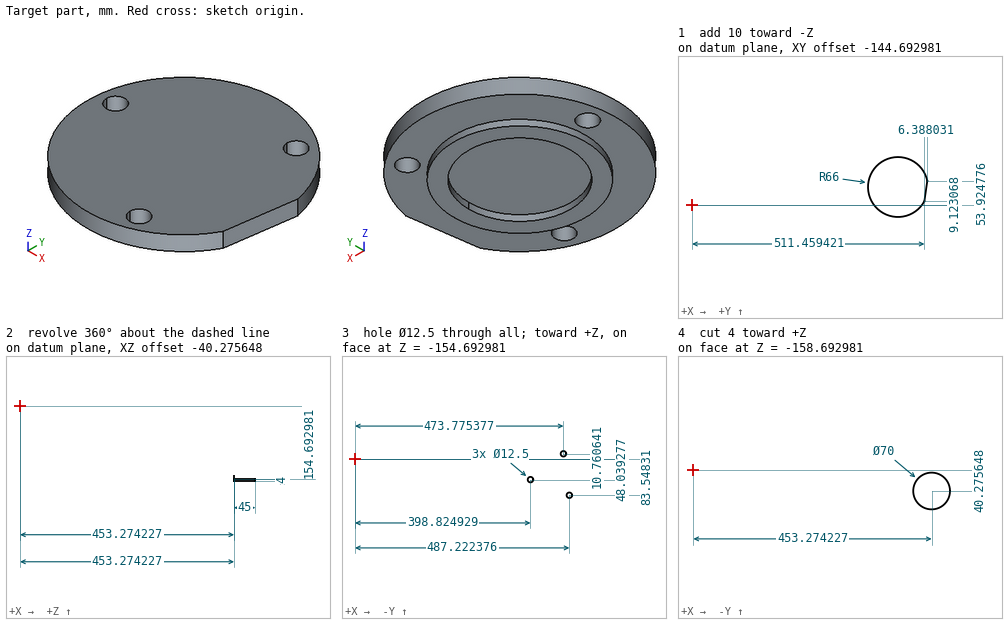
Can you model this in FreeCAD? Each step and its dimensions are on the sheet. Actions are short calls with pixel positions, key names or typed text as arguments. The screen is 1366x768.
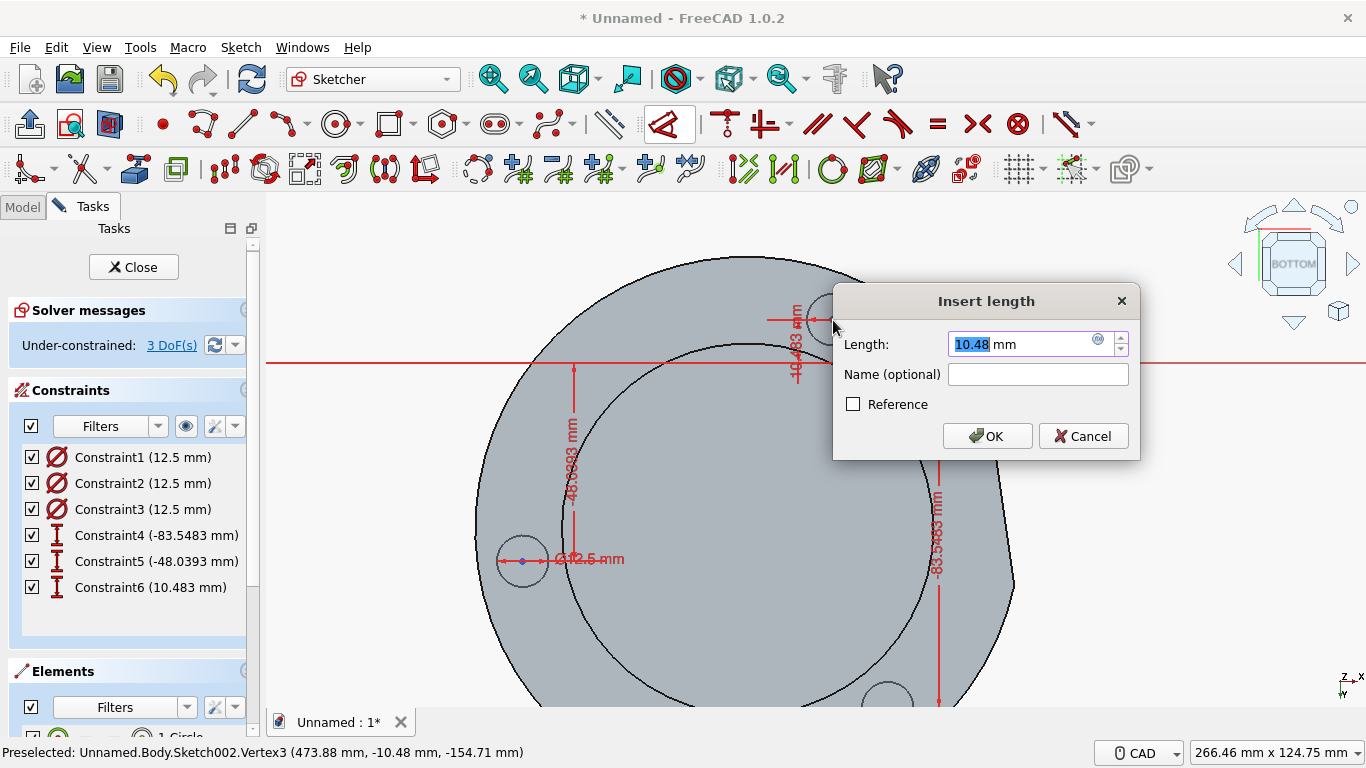
text(10.760641)
key(Return)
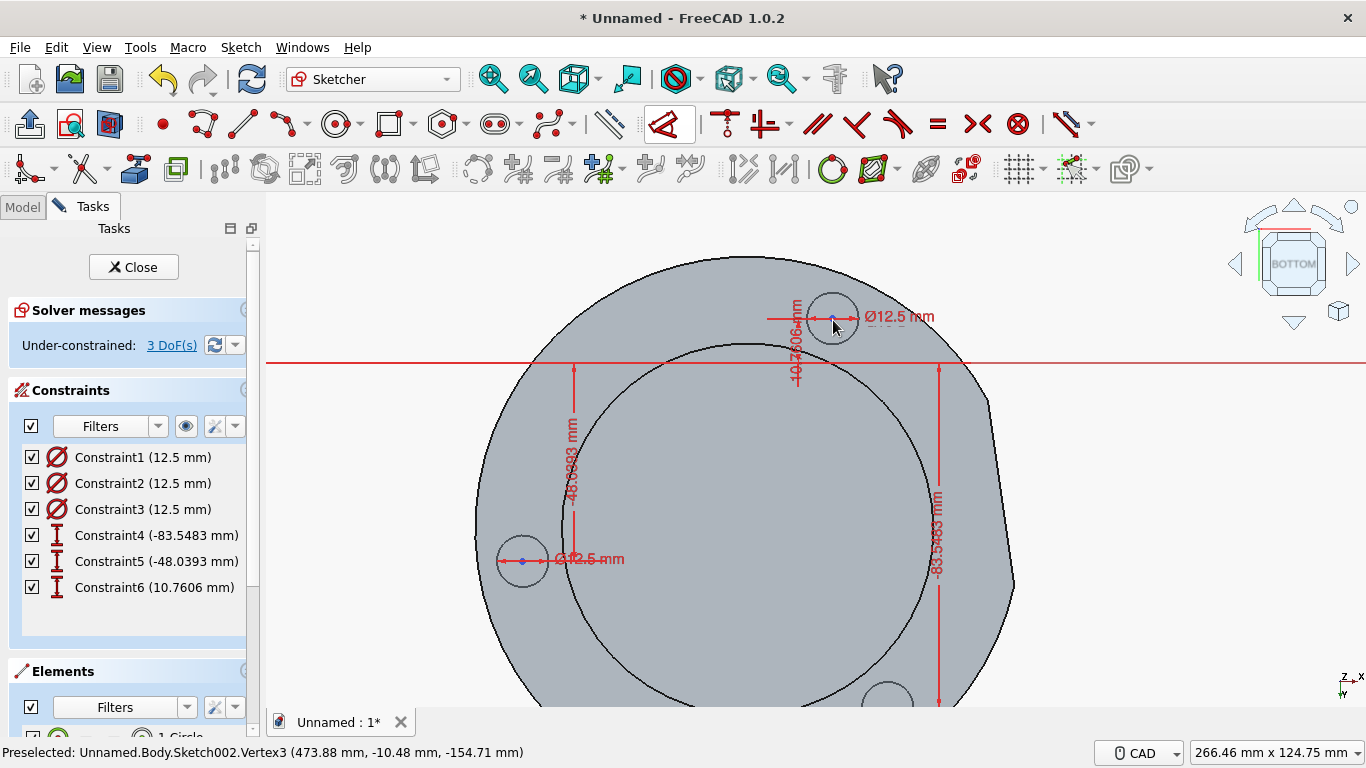
click(523, 561)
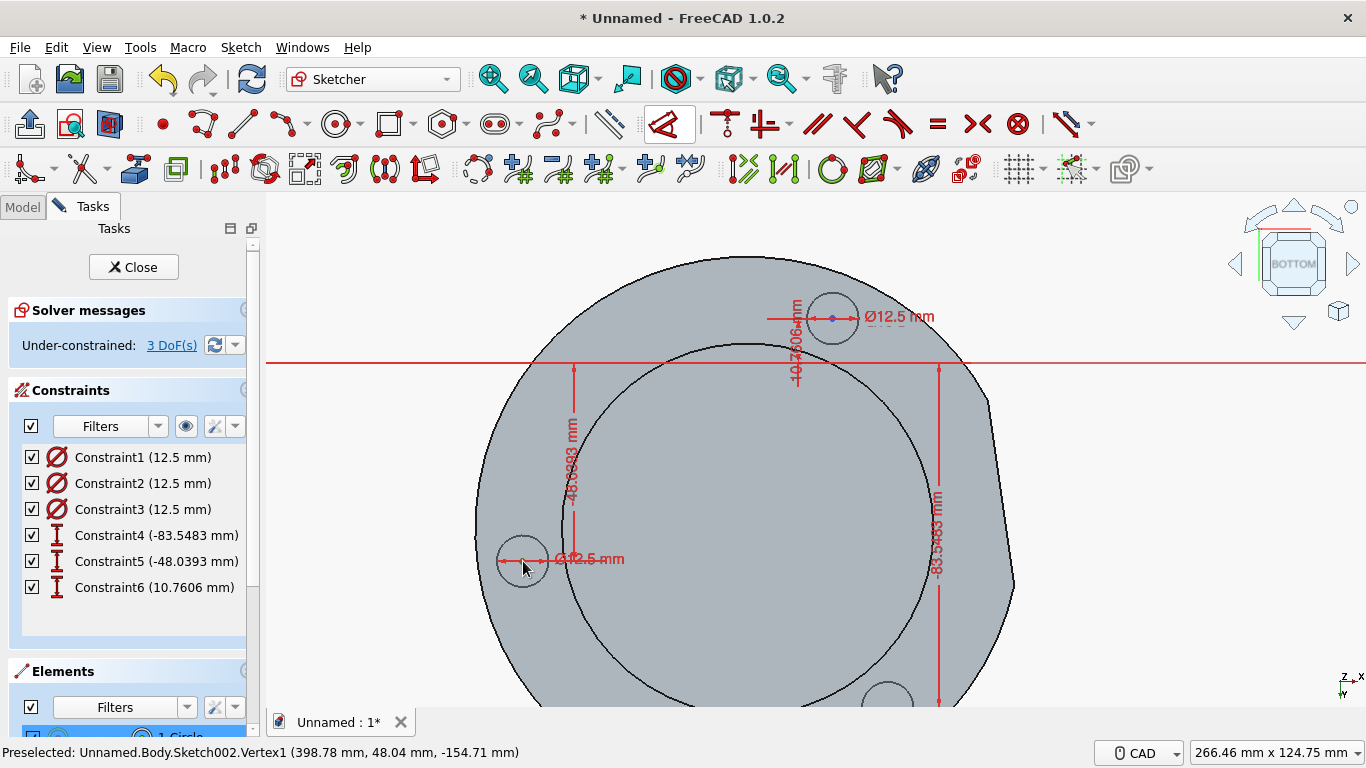
key(l)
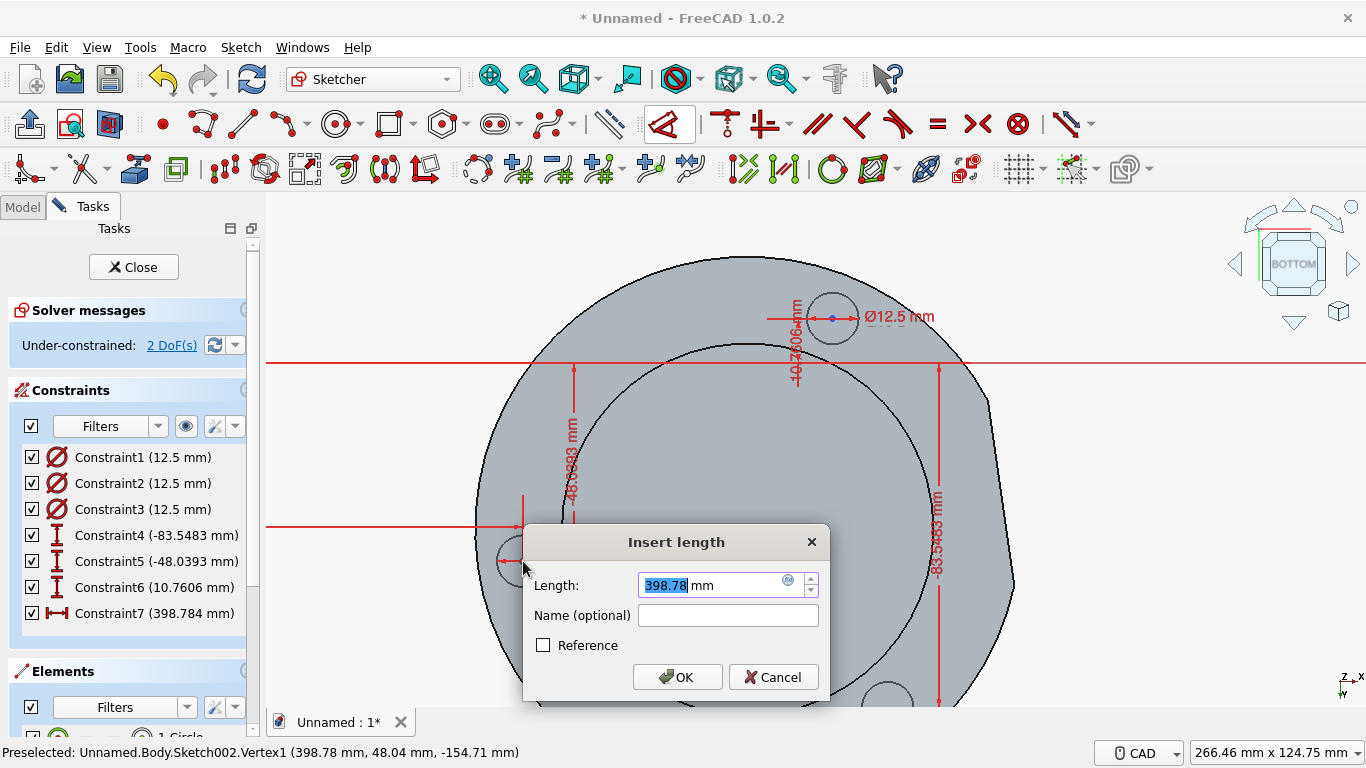
text(398.824929)
key(Return)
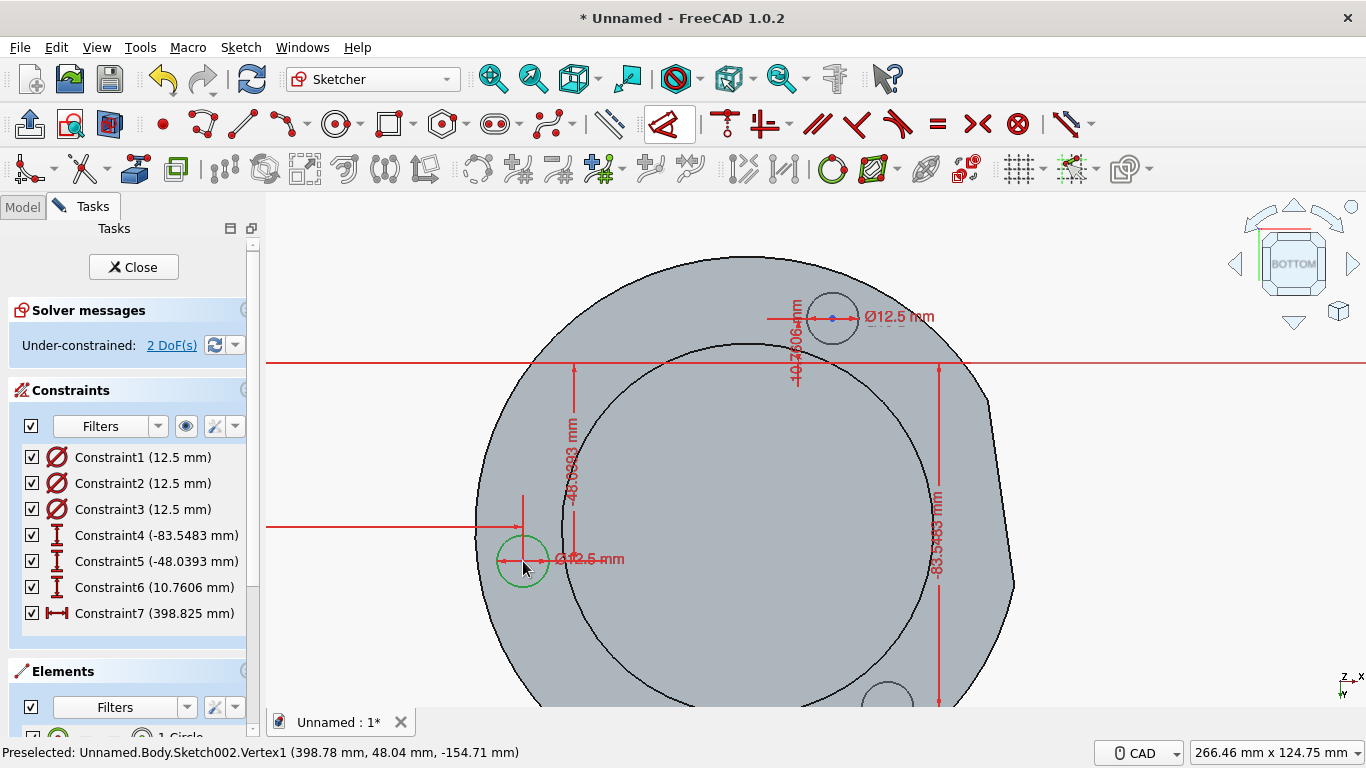
scroll(833, 320, down, 2)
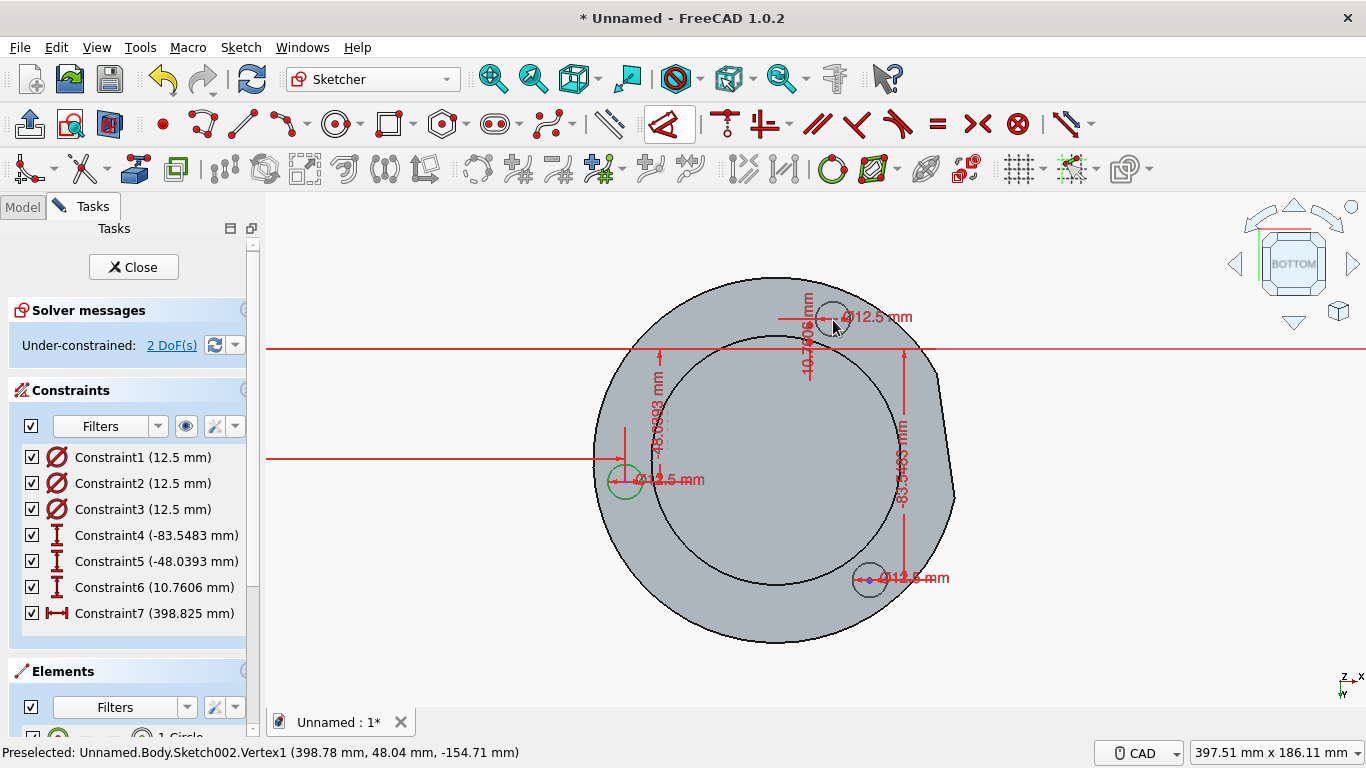
click(870, 580)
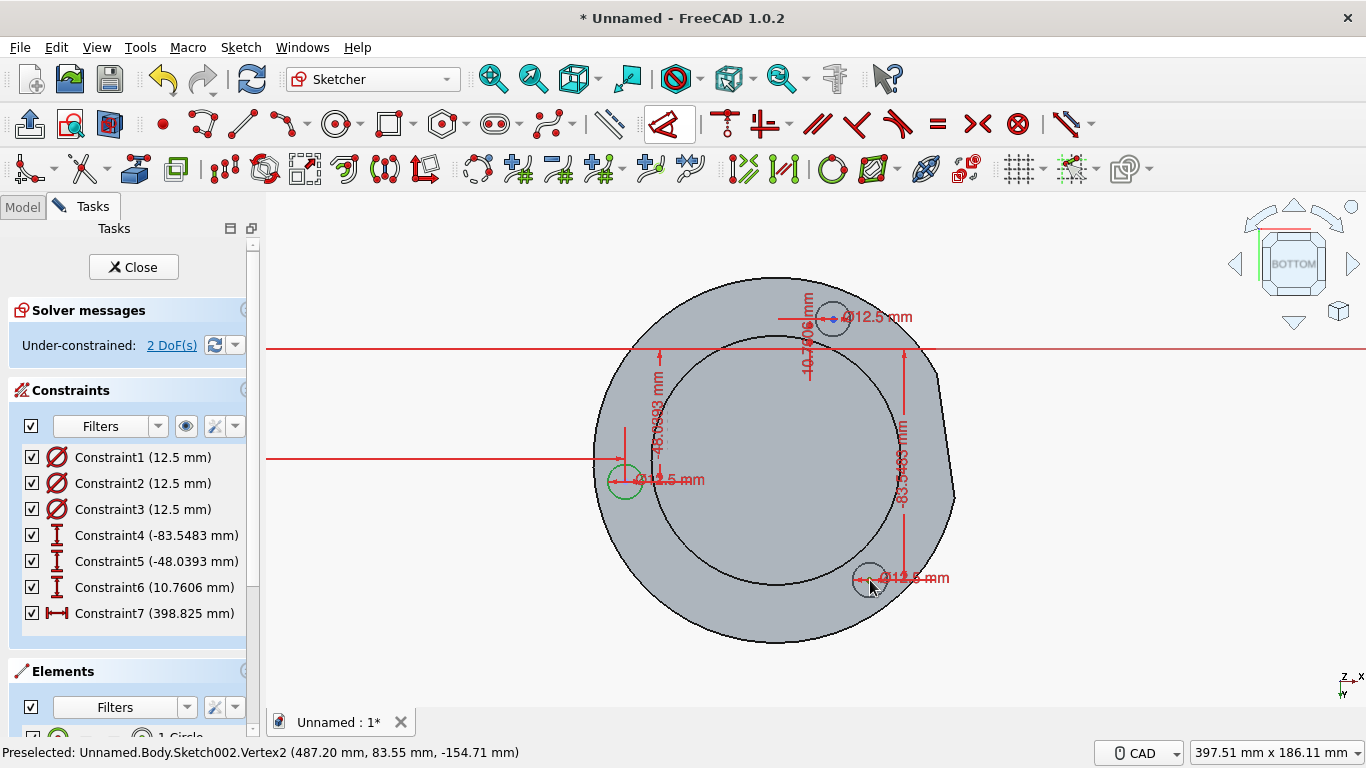
key(l)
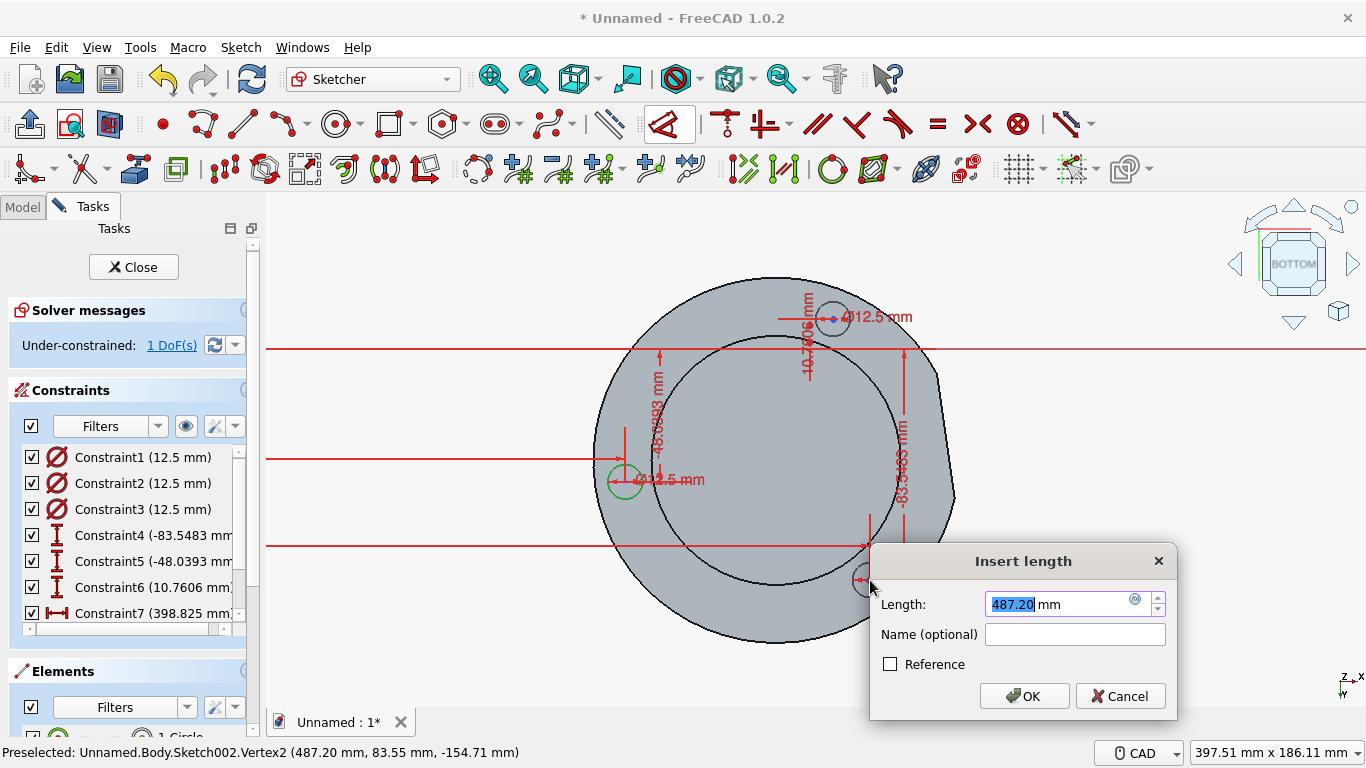
text(487.222376)
key(Return)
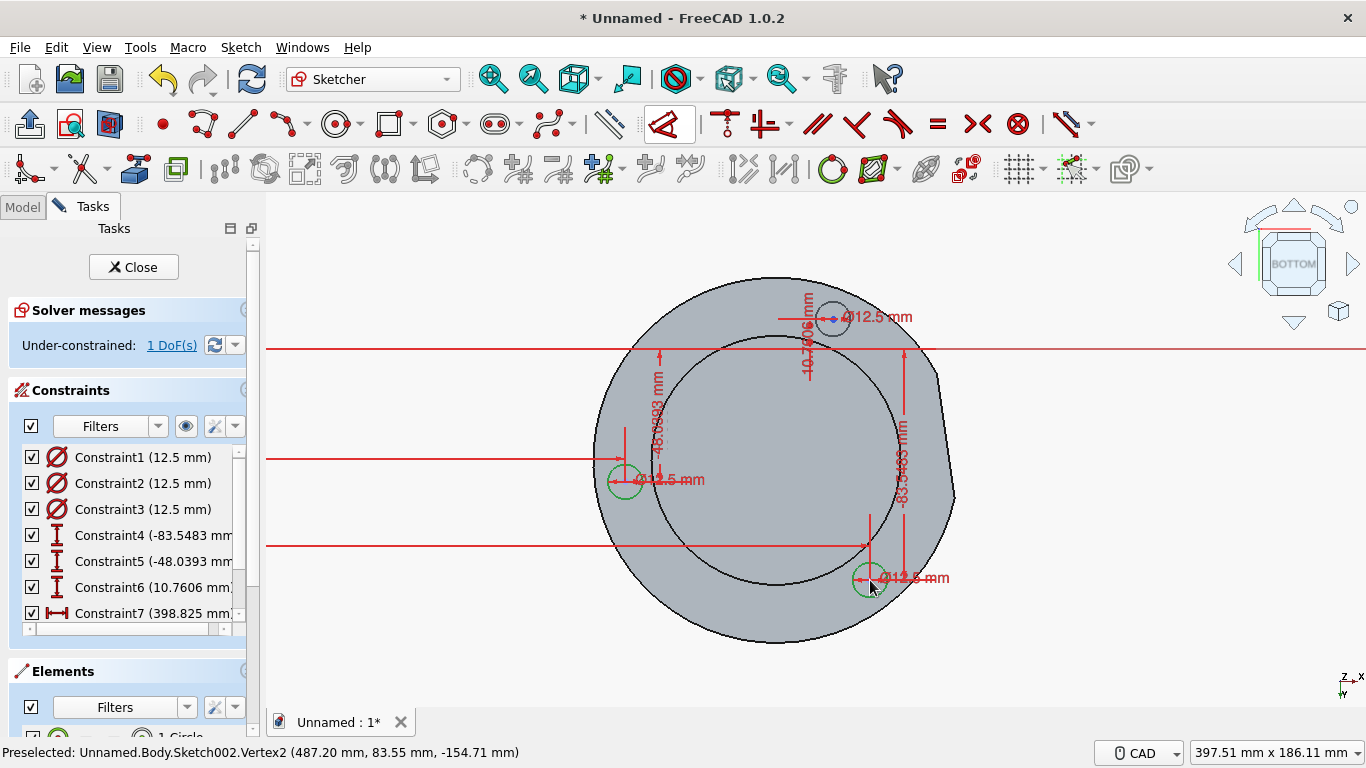
click(833, 319)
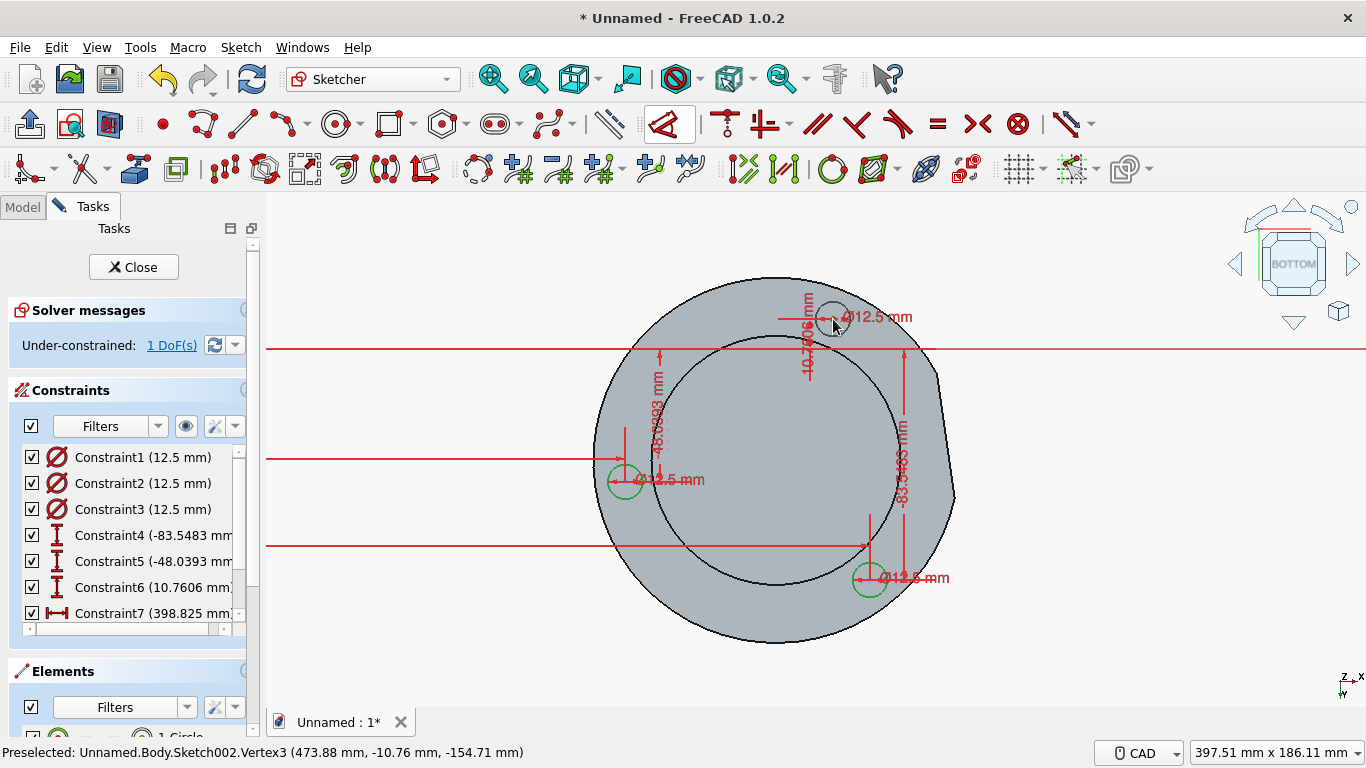
key(l)